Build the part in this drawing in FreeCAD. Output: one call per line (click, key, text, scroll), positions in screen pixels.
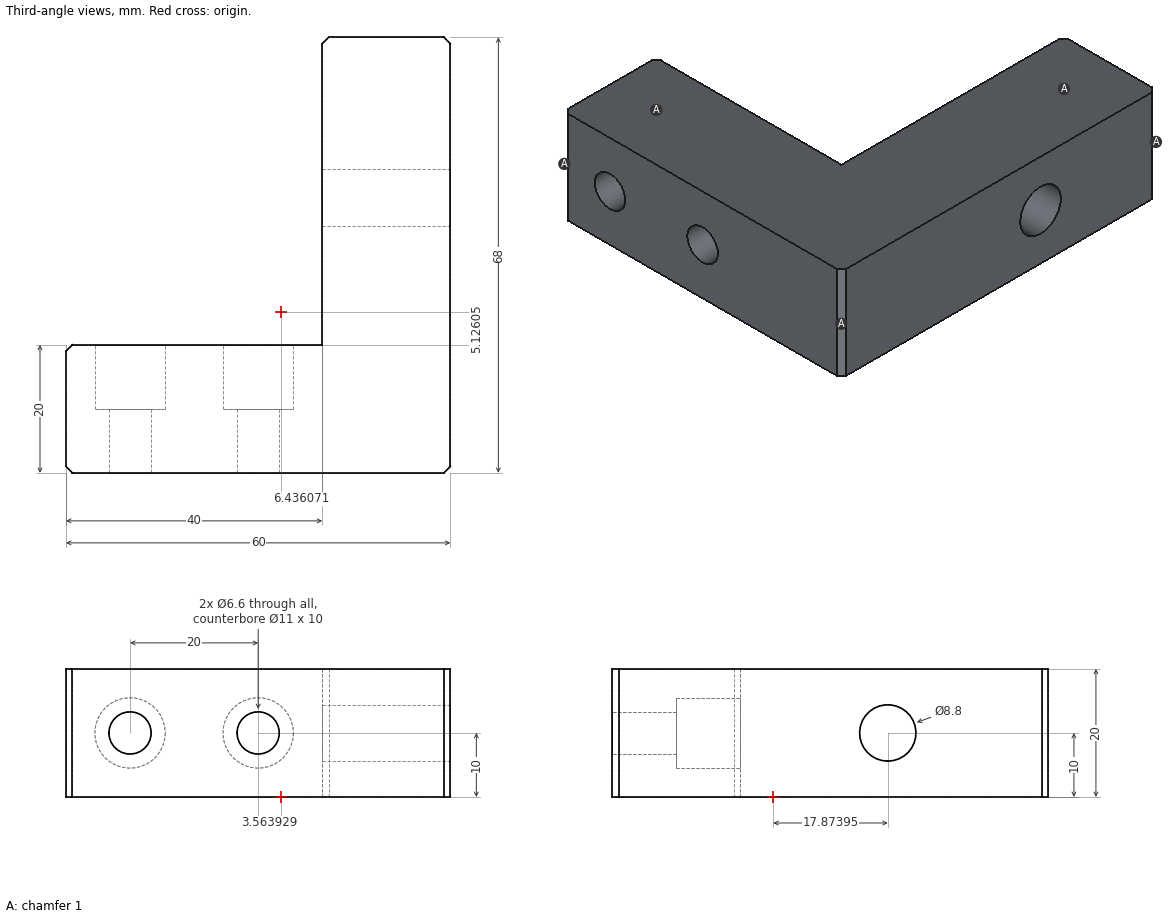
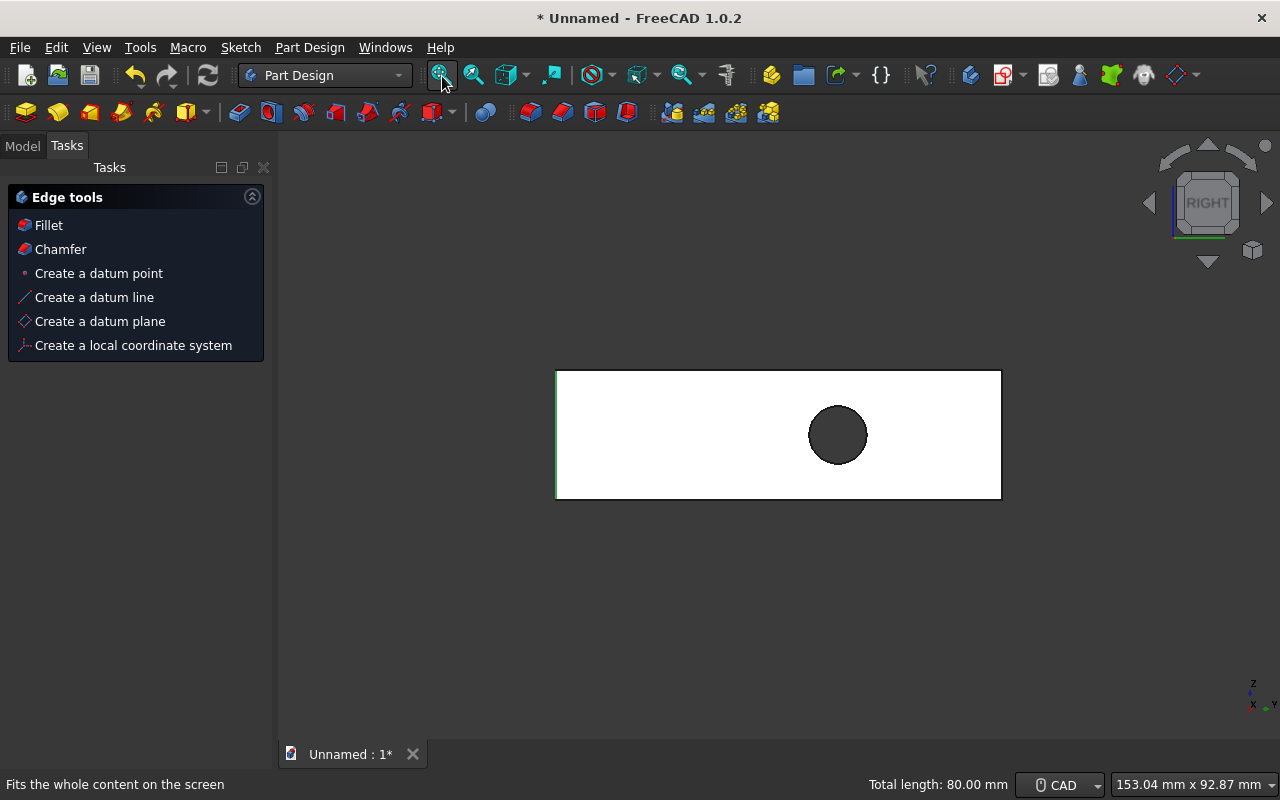
click(1002, 434, ctrl)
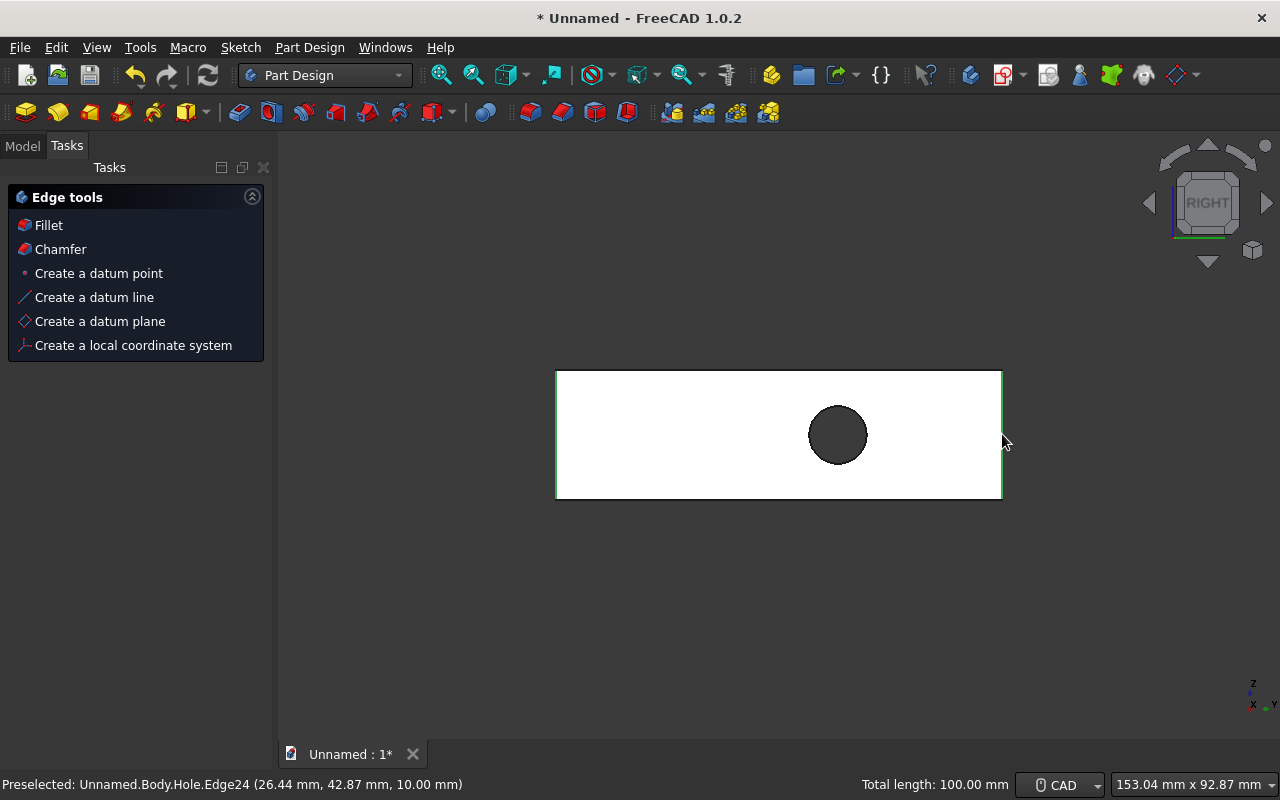
click(564, 112)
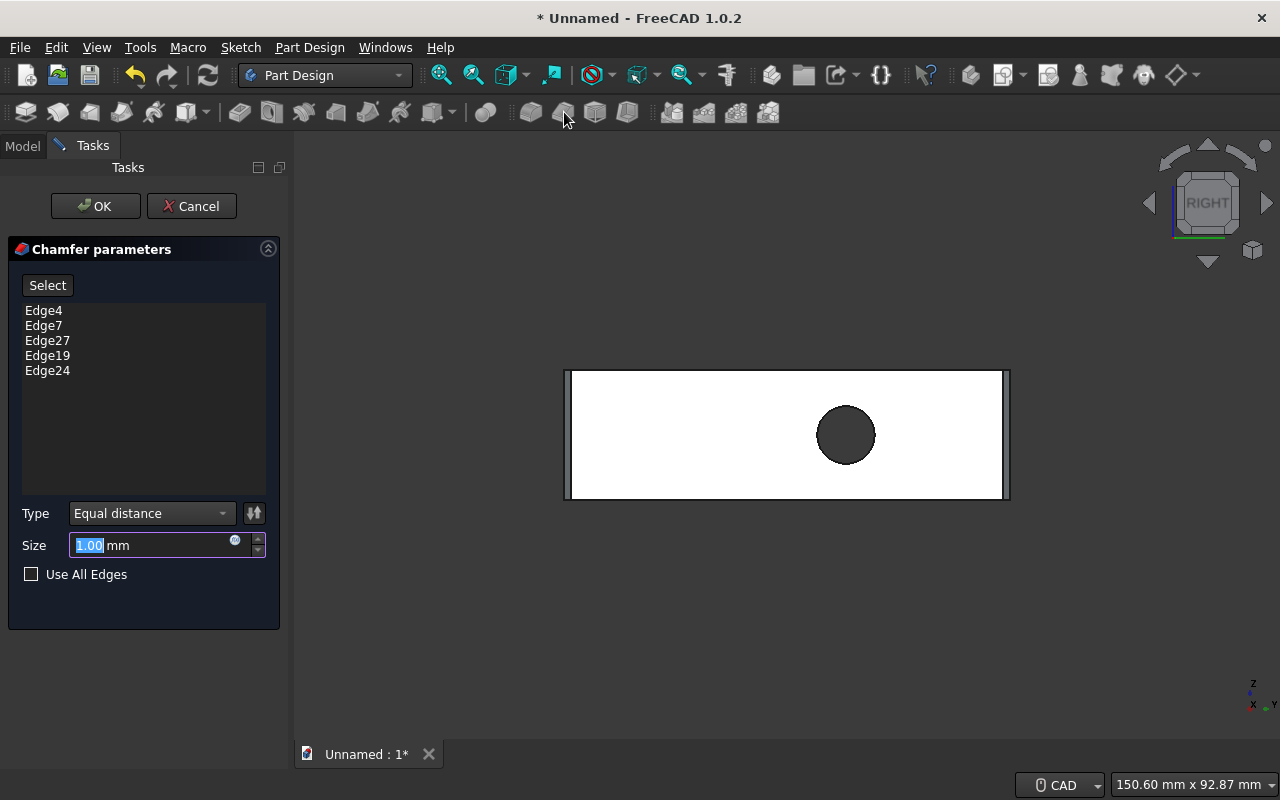
text(1)
key(Tab)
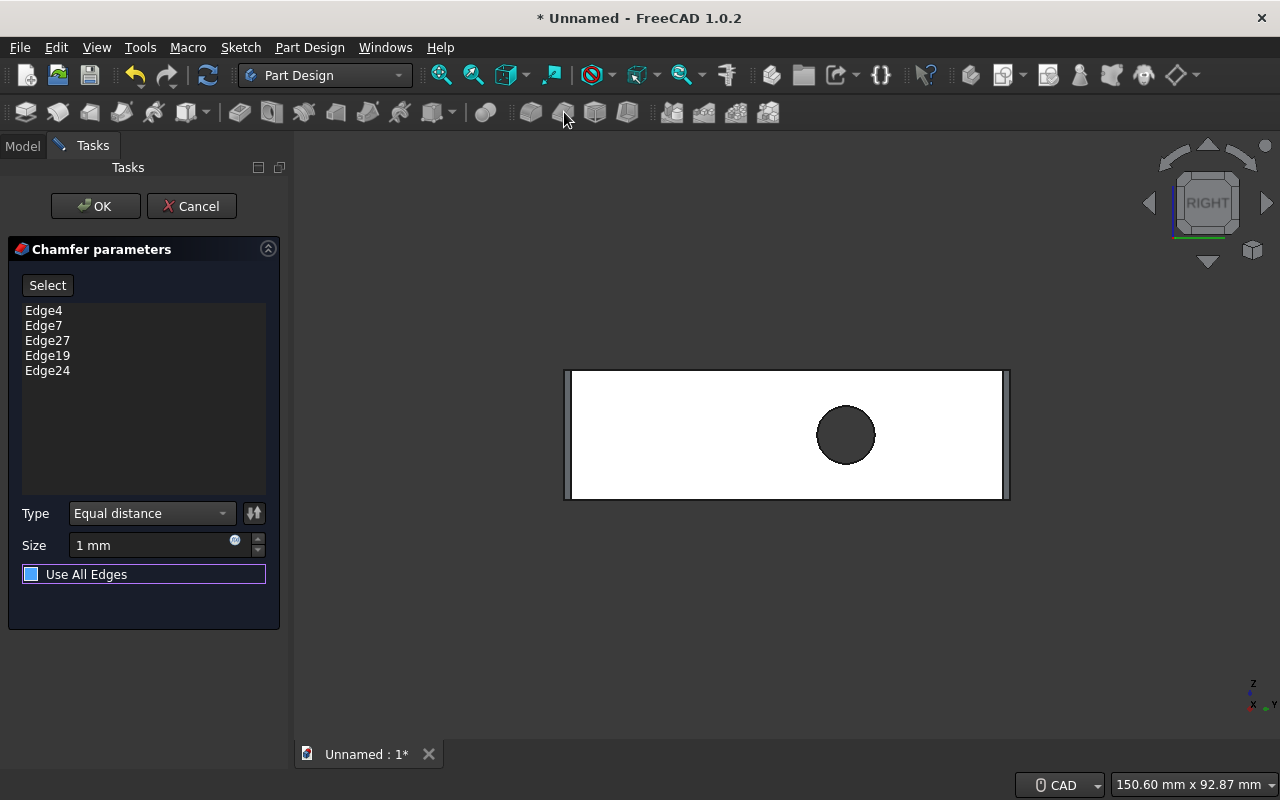
click(96, 206)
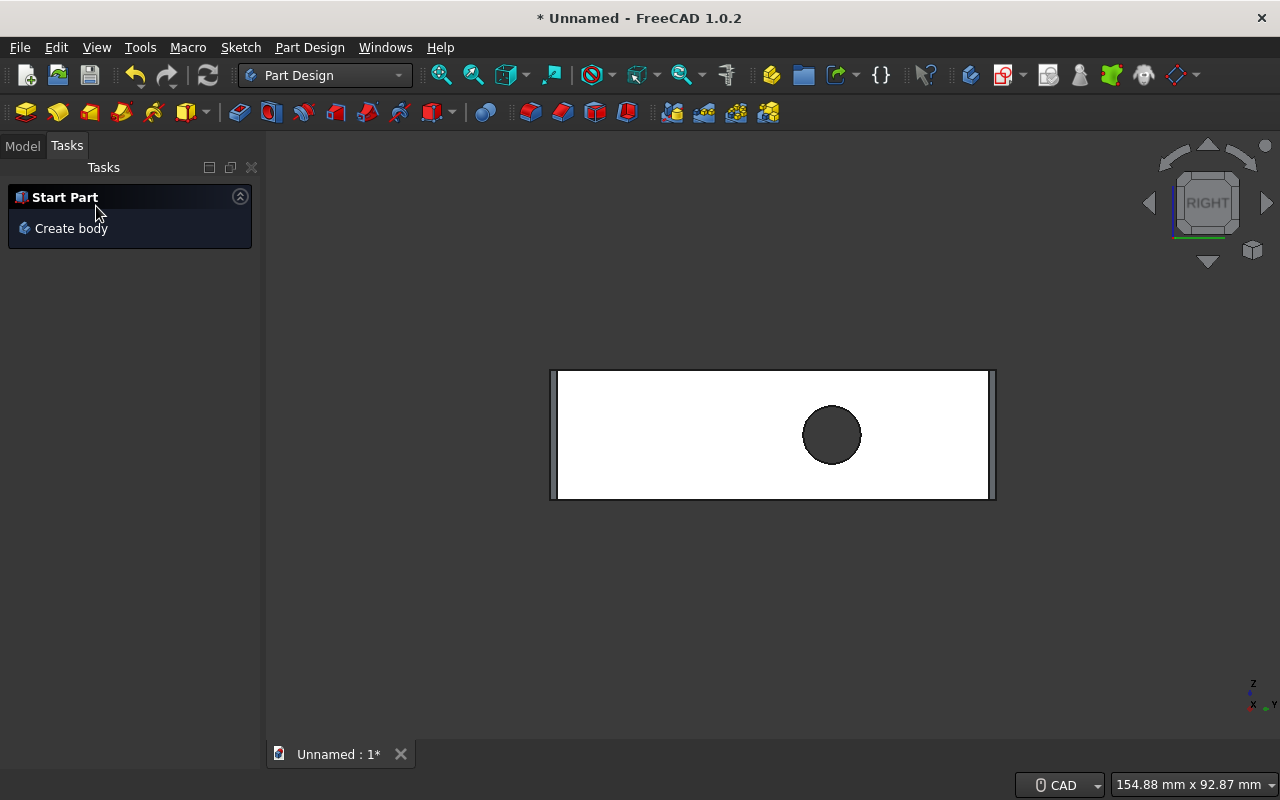
key(0)